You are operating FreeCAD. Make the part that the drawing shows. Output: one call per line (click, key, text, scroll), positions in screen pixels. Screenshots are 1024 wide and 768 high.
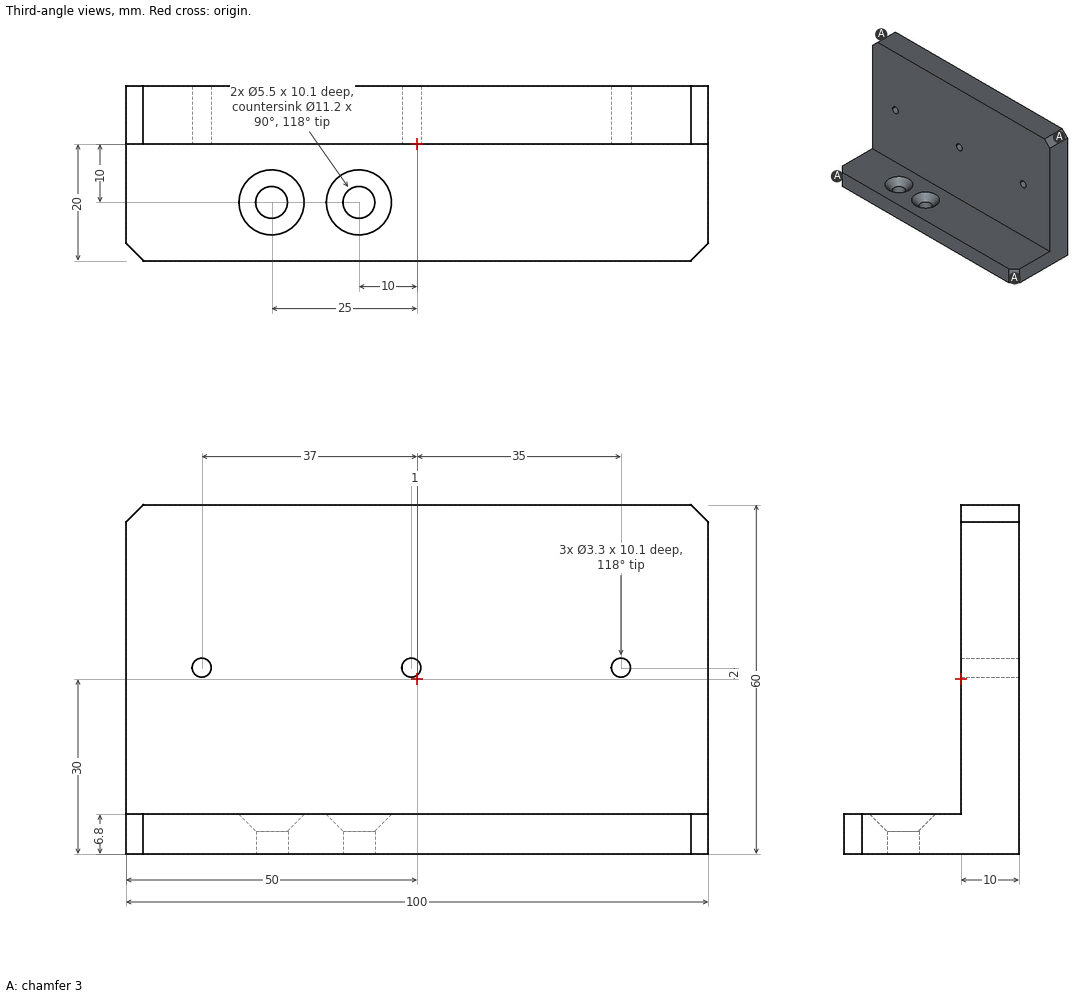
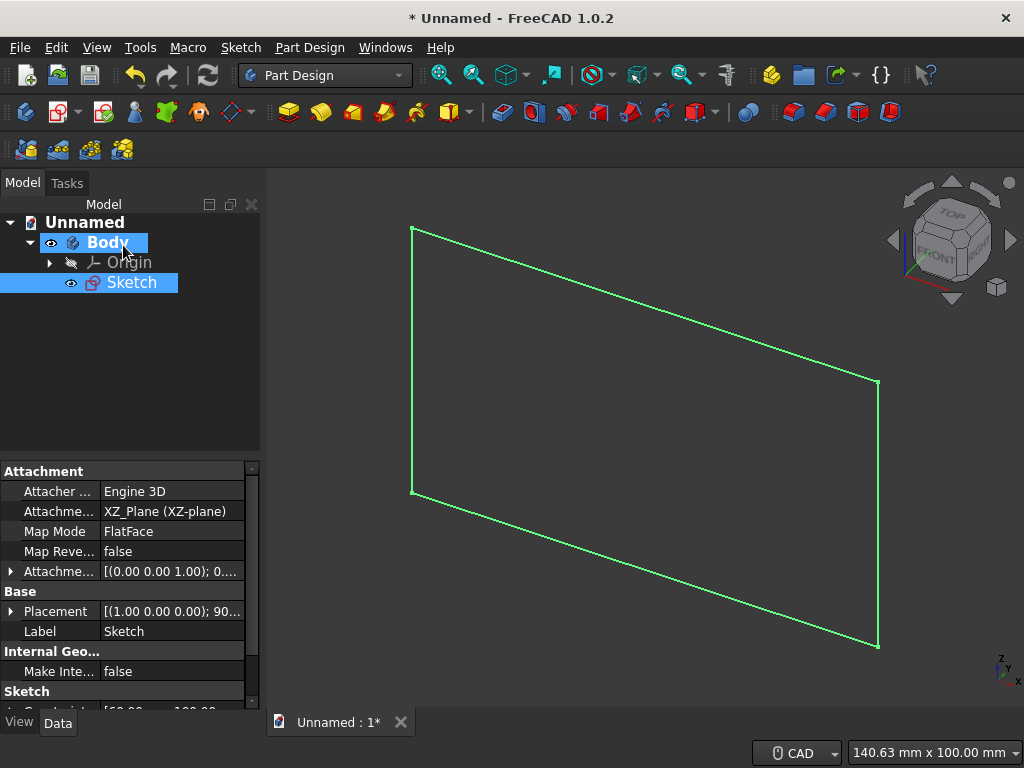
click(290, 112)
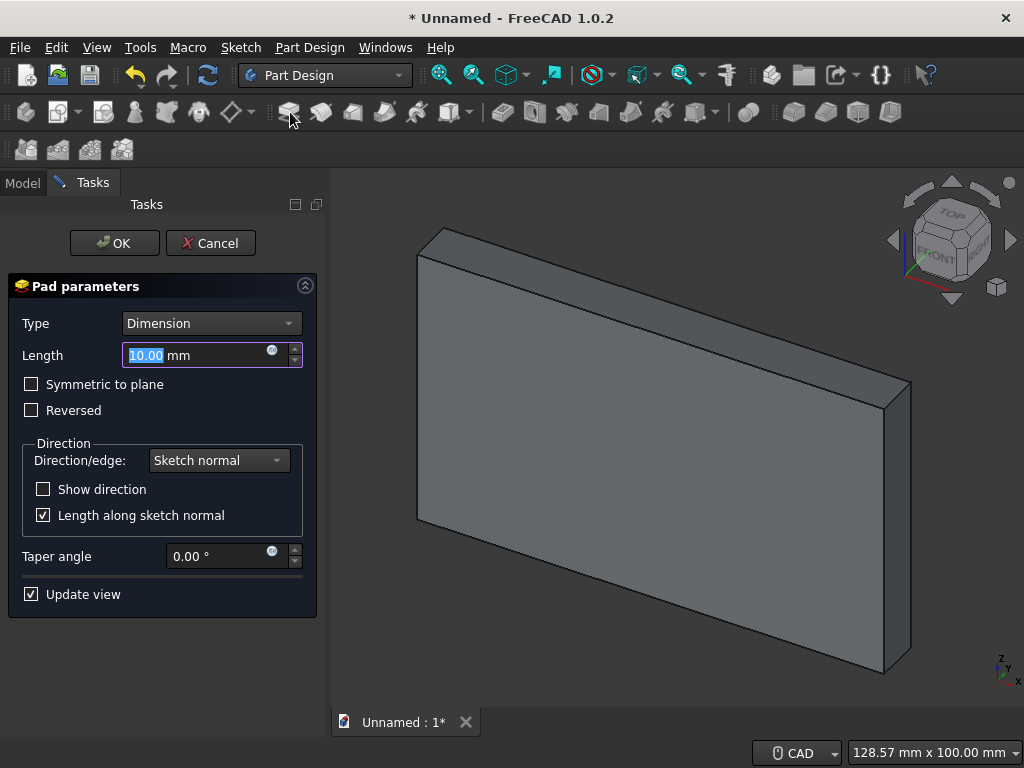
text(10)
key(Tab)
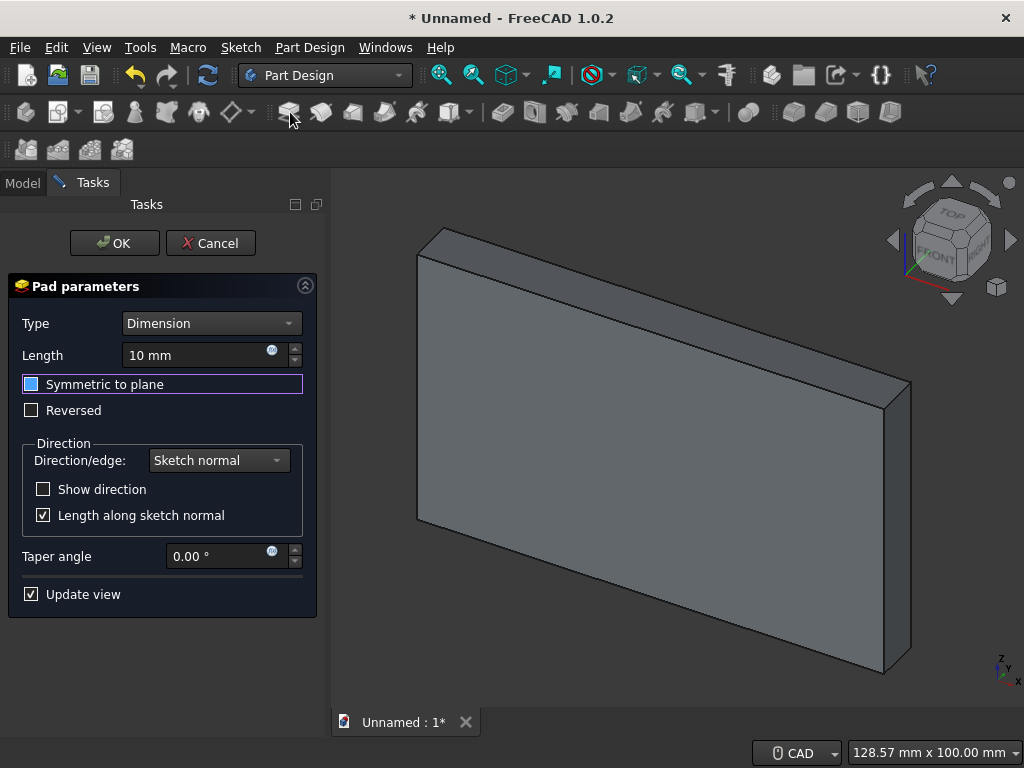
click(30, 410)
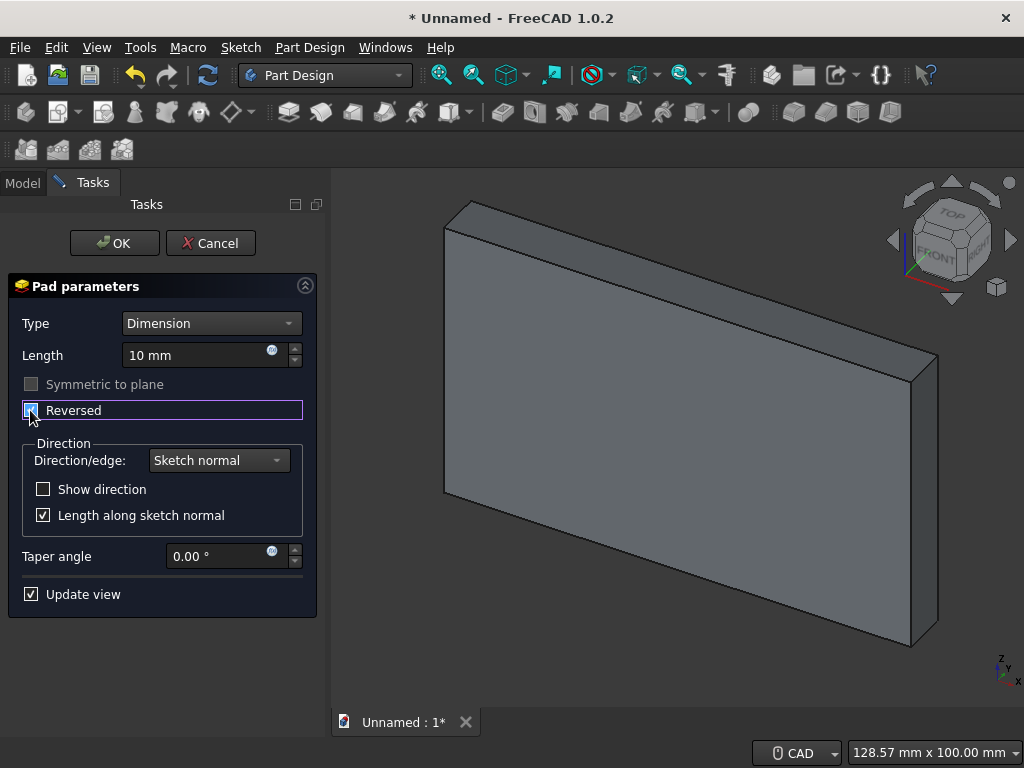
click(115, 243)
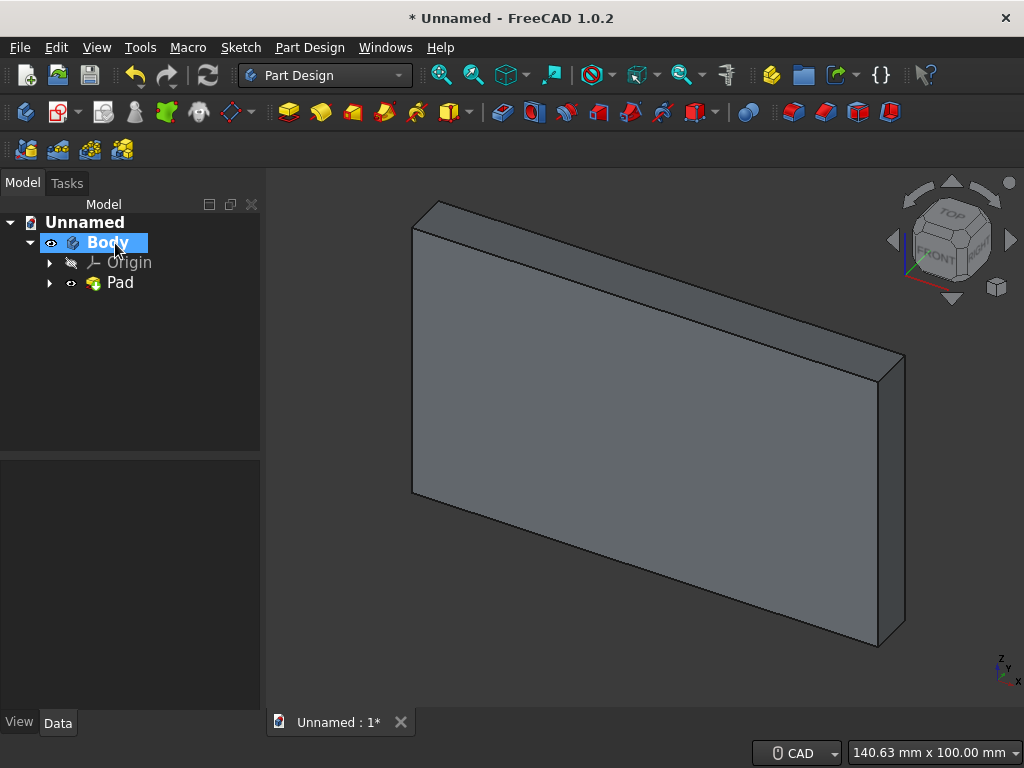
click(58, 112)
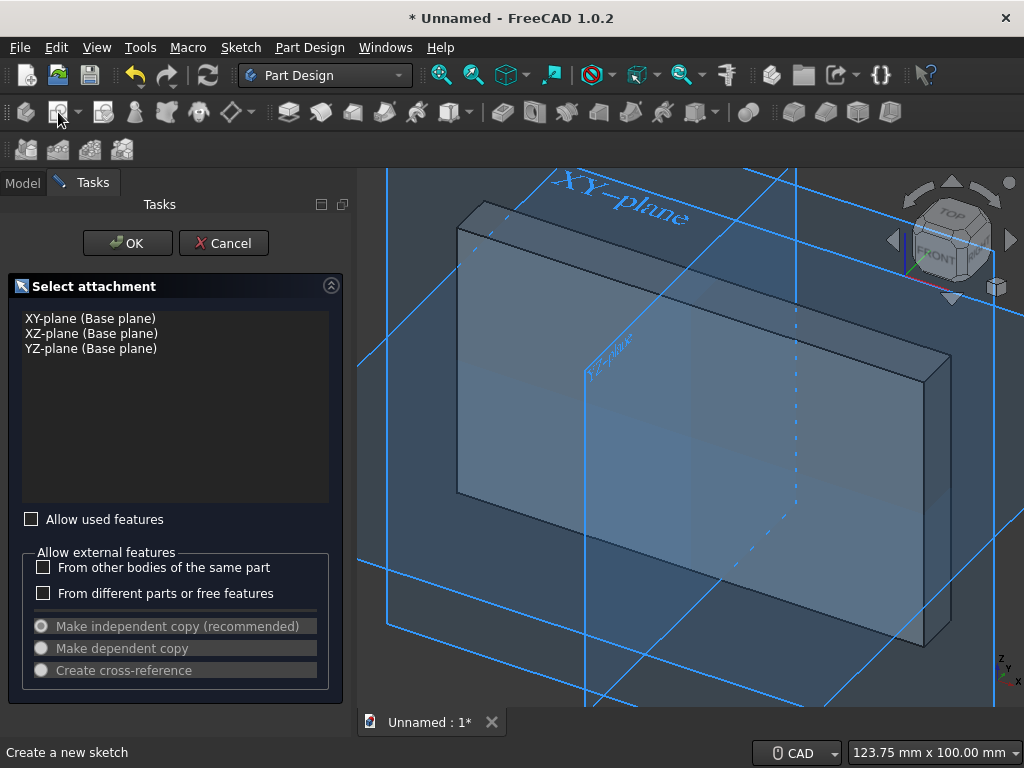
click(82, 334)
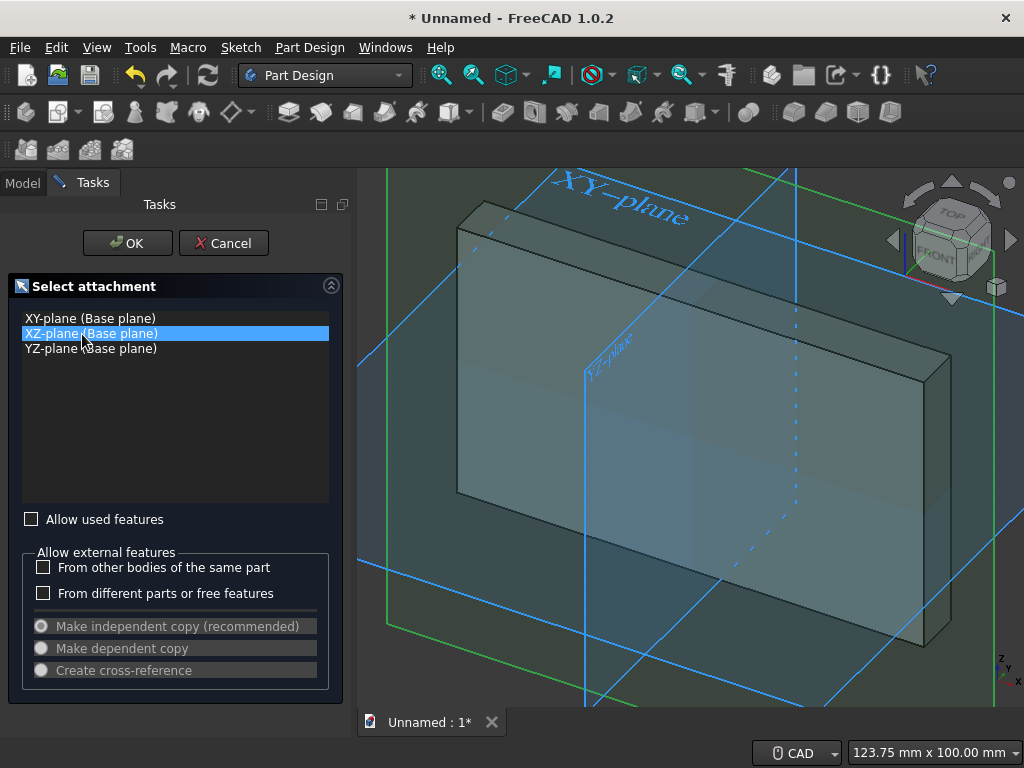
click(128, 243)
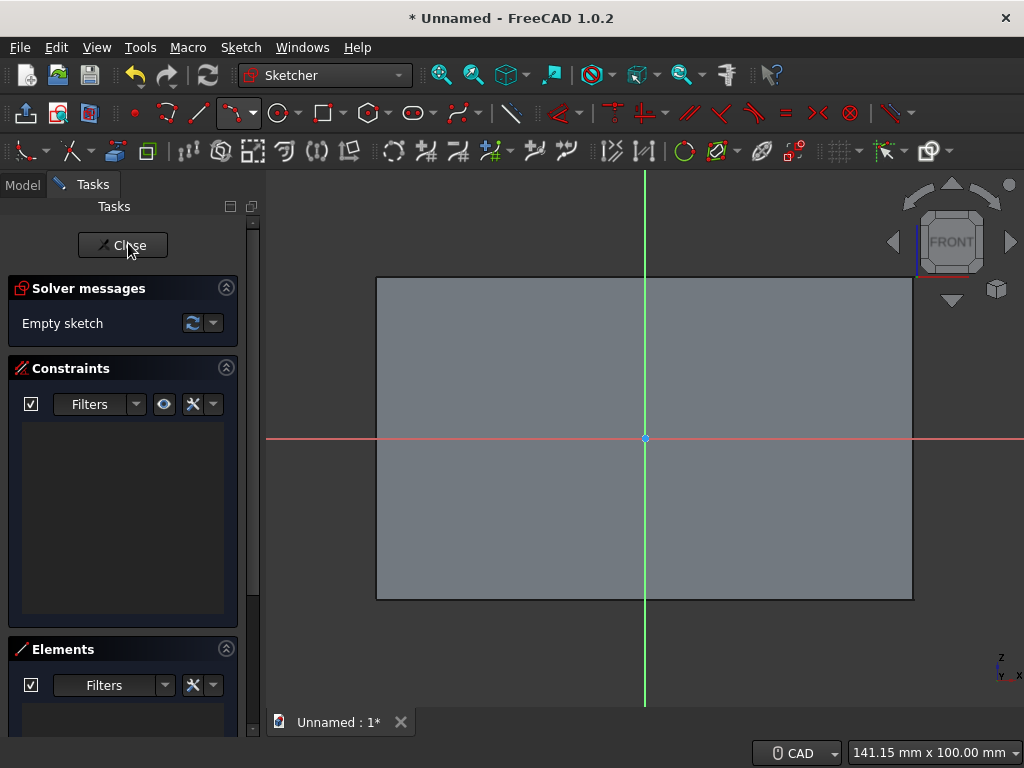
scroll(294, 198, down, 1)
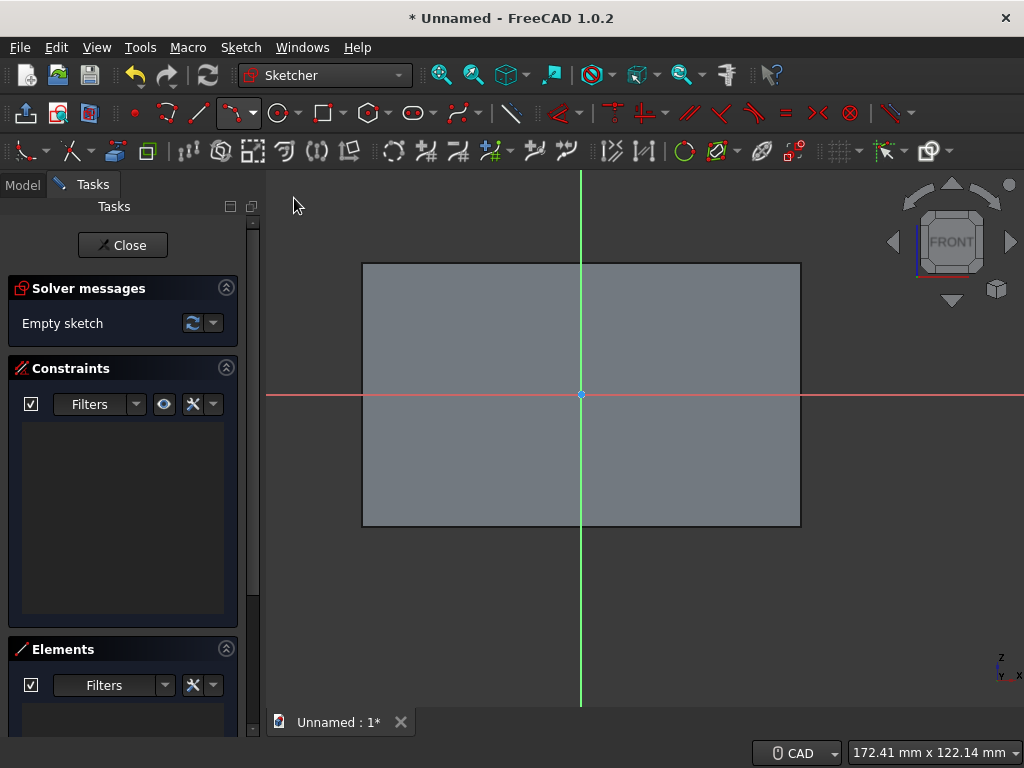
key(g)
key(r)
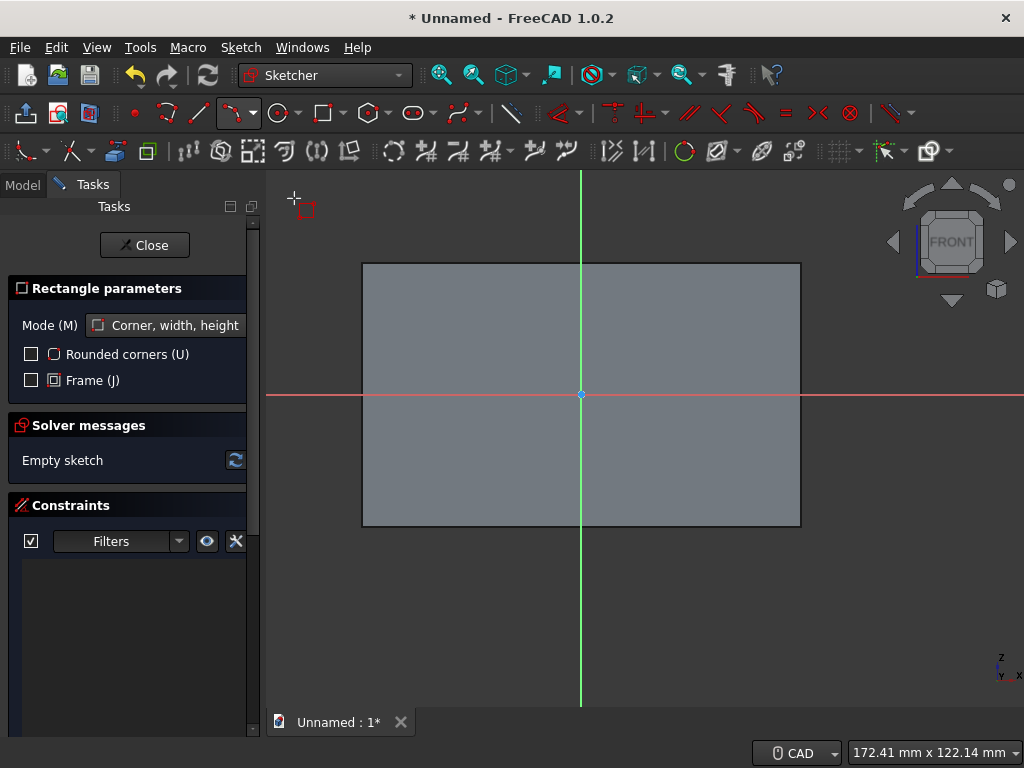
click(362, 497)
click(801, 527)
key(Escape)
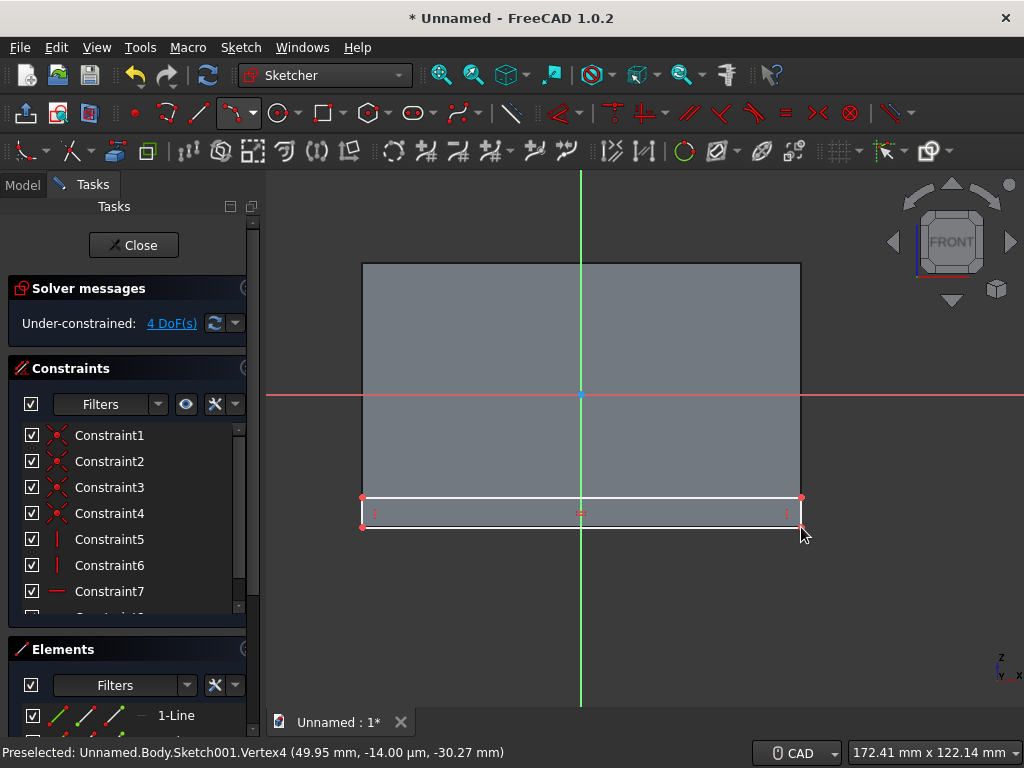
key(d)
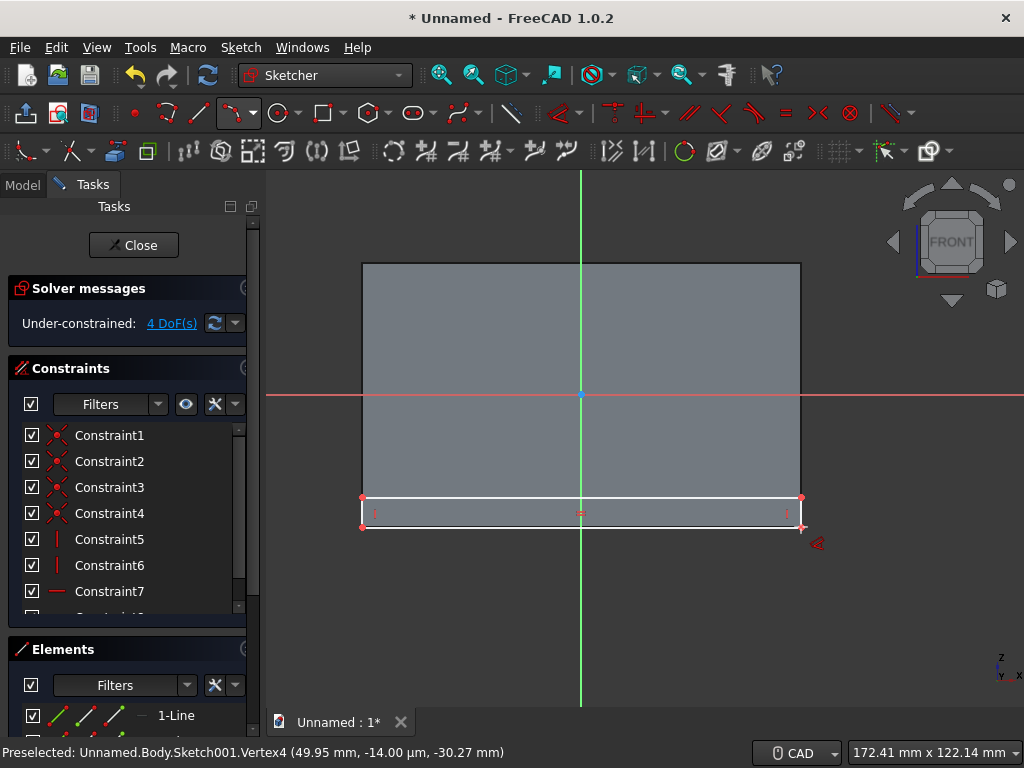
scroll(362, 510, up, 2)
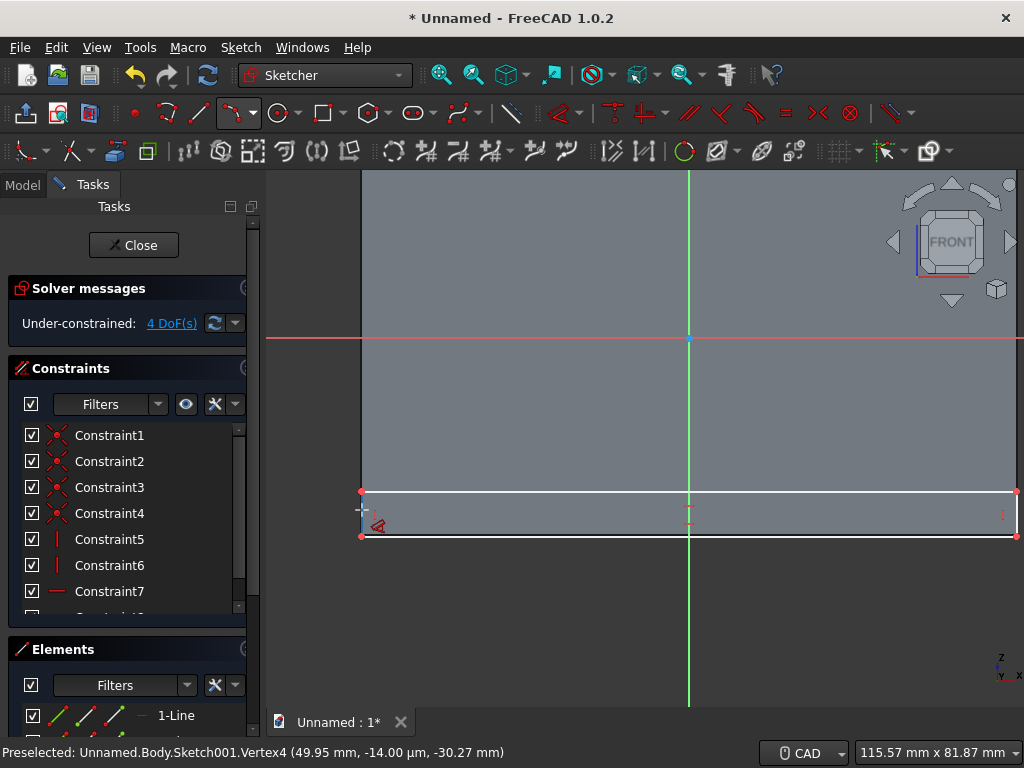
click(362, 510)
click(328, 514)